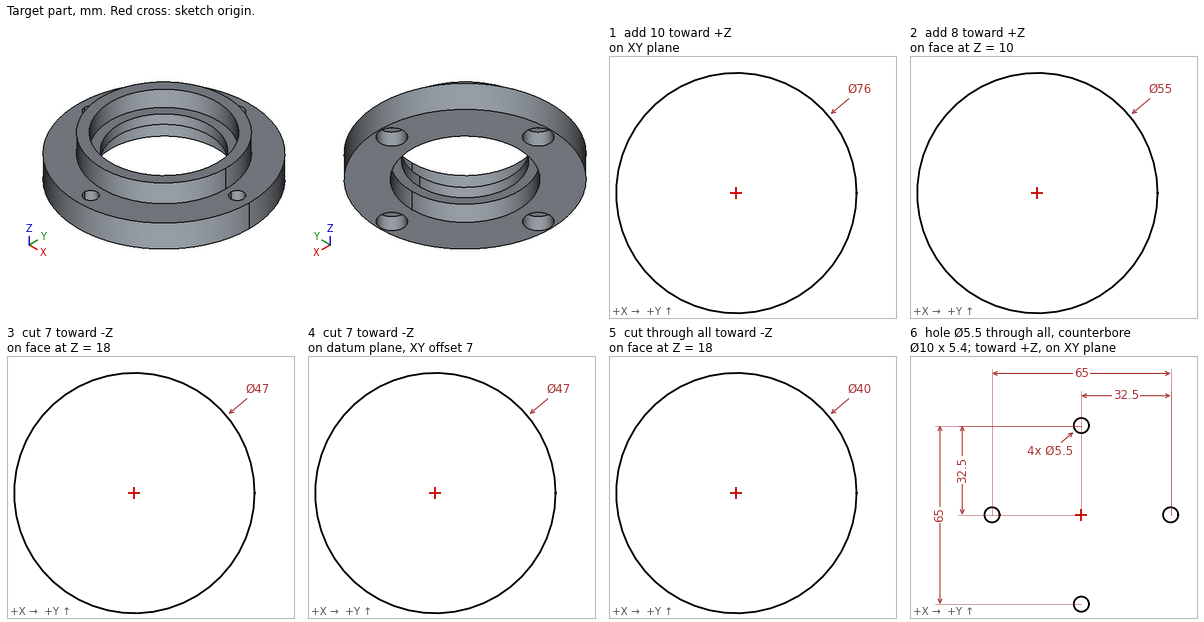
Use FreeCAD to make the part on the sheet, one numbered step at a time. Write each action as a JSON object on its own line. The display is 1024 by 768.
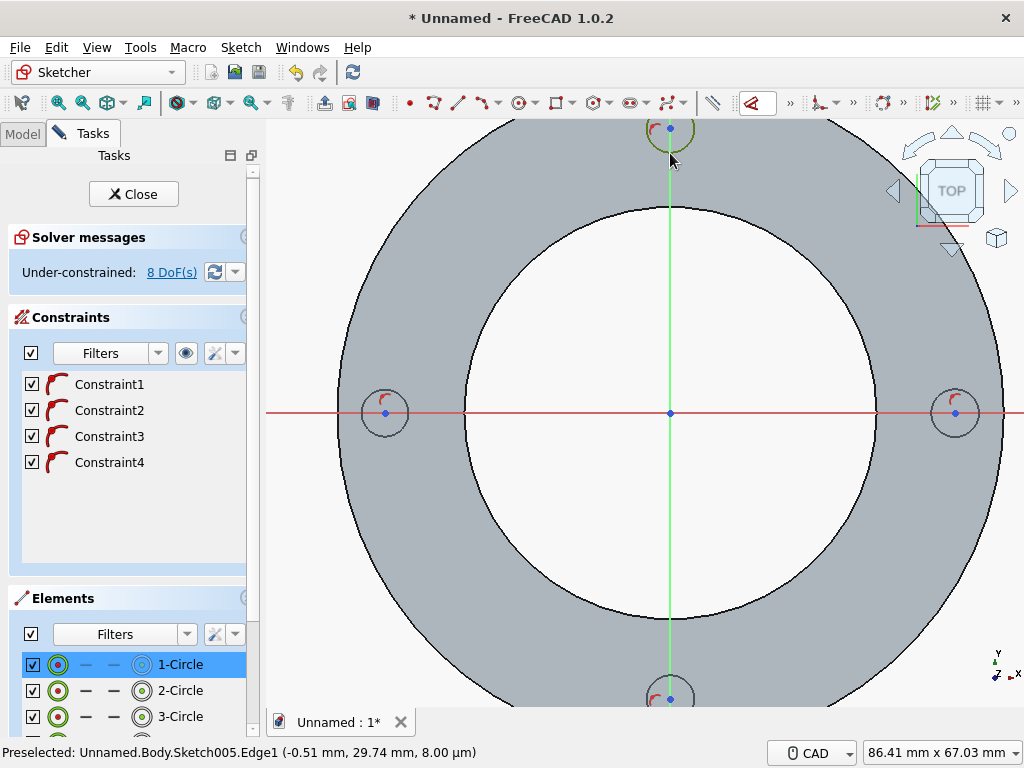
{"action": "scroll", "coordinate": [385, 413], "scroll_direction": "down", "scroll_amount": 2}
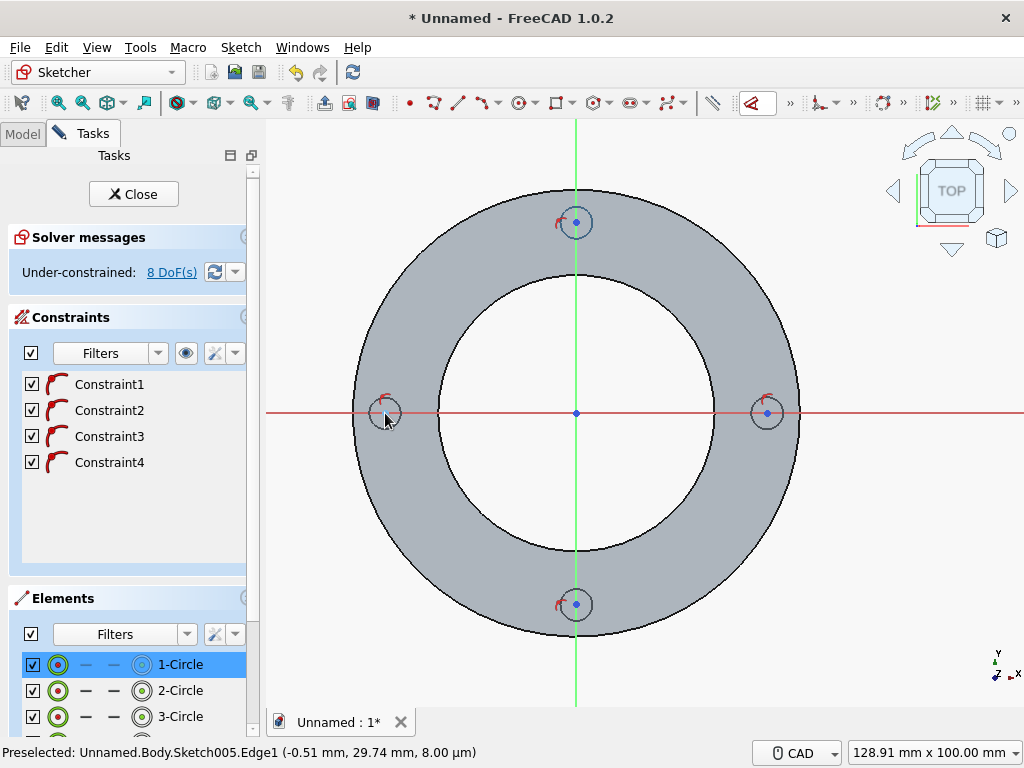
{"action": "left_click", "coordinate": [778, 402]}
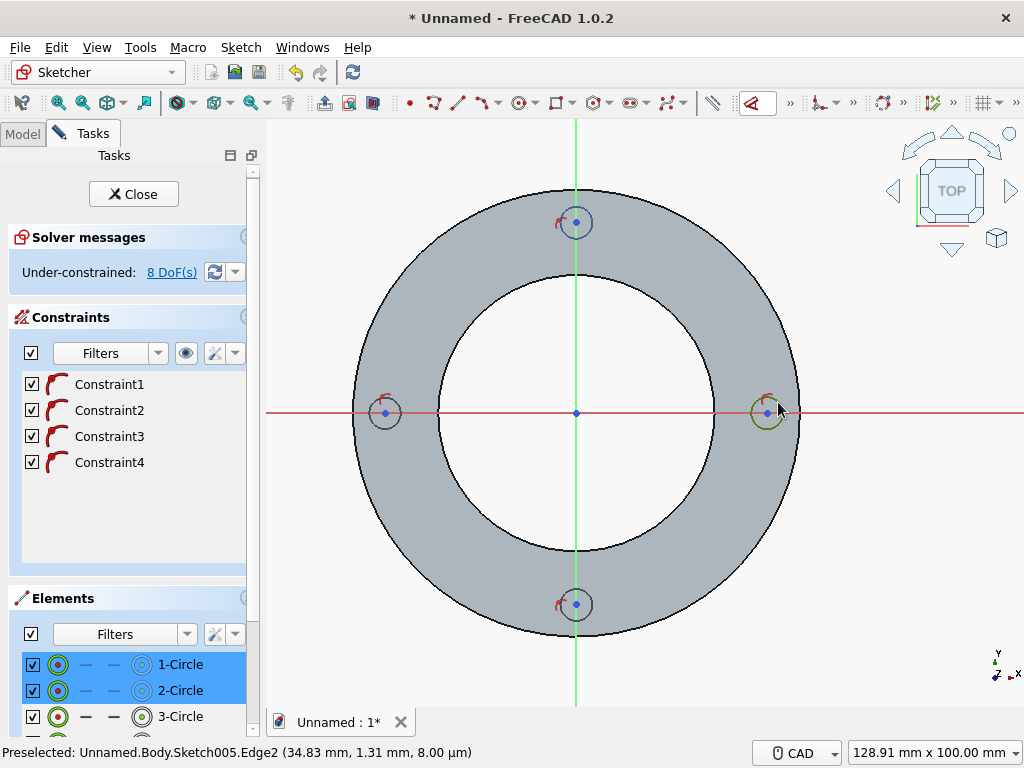
{"action": "scroll", "coordinate": [588, 594], "scroll_direction": "up", "scroll_amount": 2}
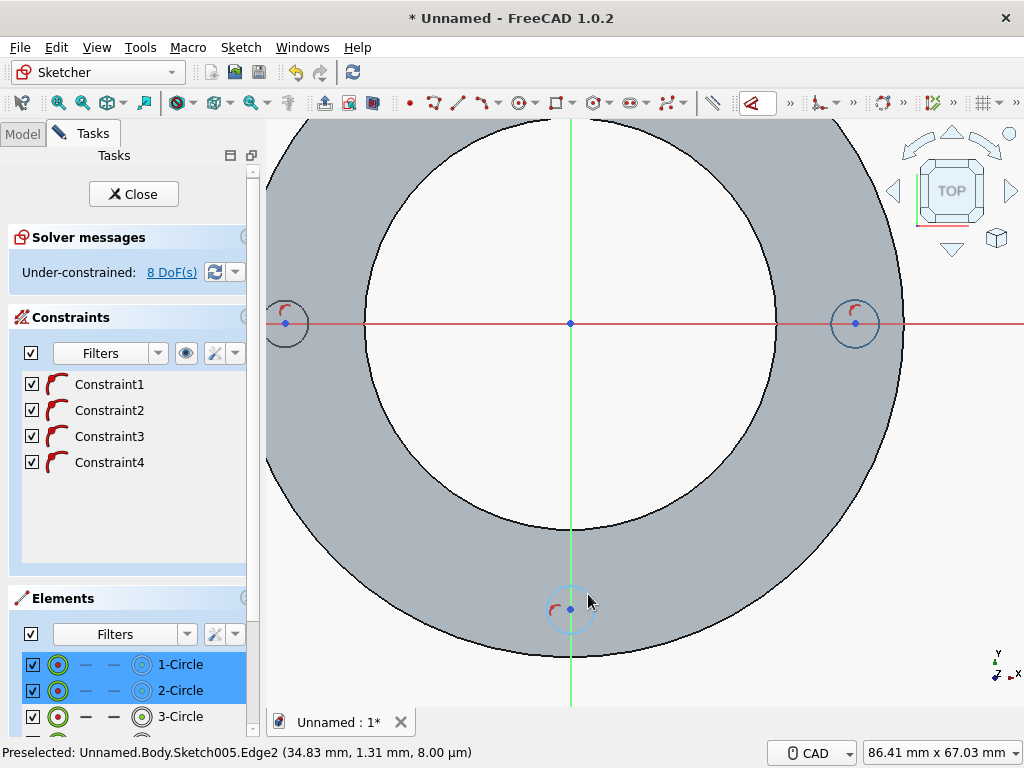
{"action": "left_click", "coordinate": [587, 593]}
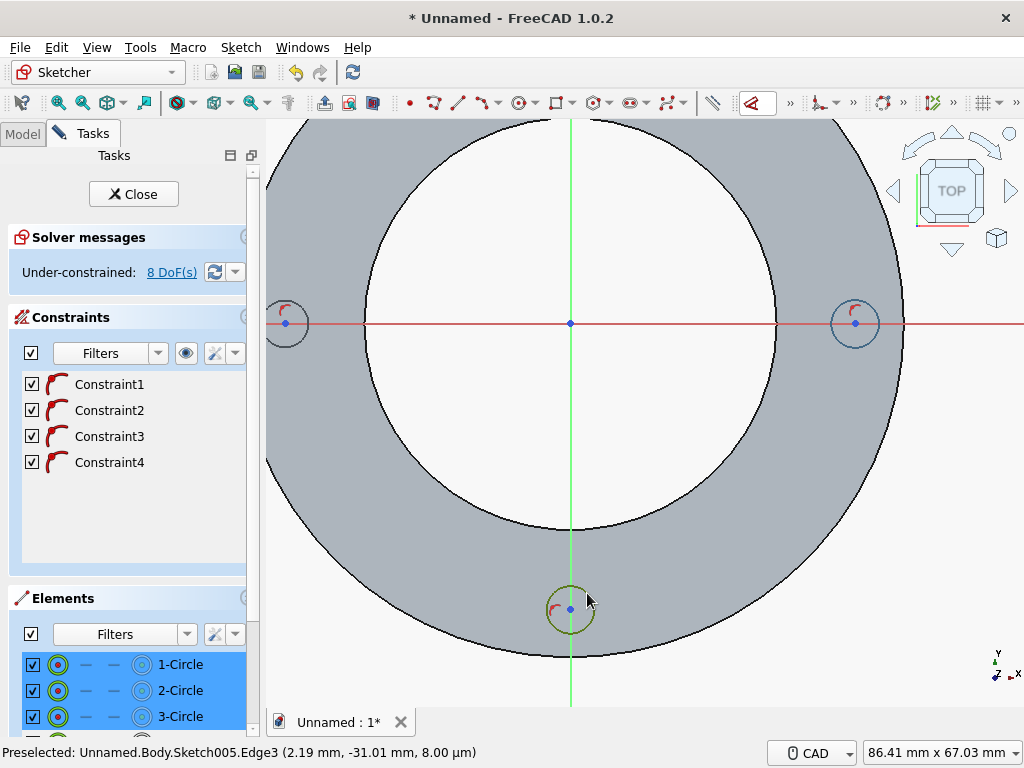
{"action": "left_click", "coordinate": [302, 307]}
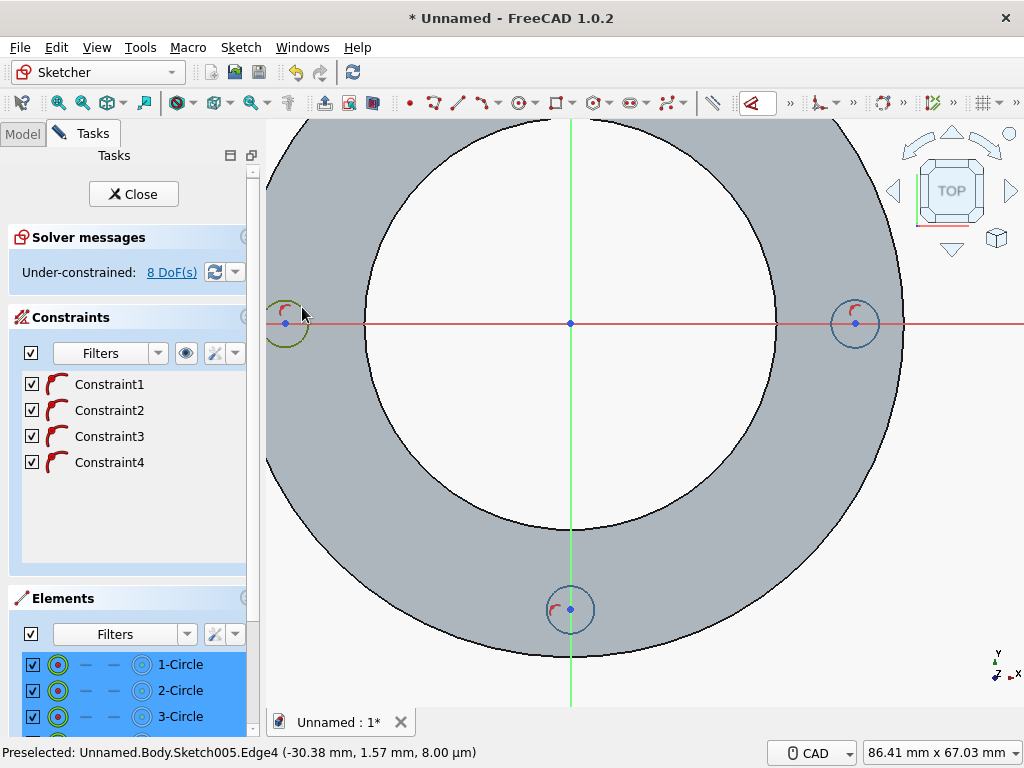
{"action": "key", "text": "e"}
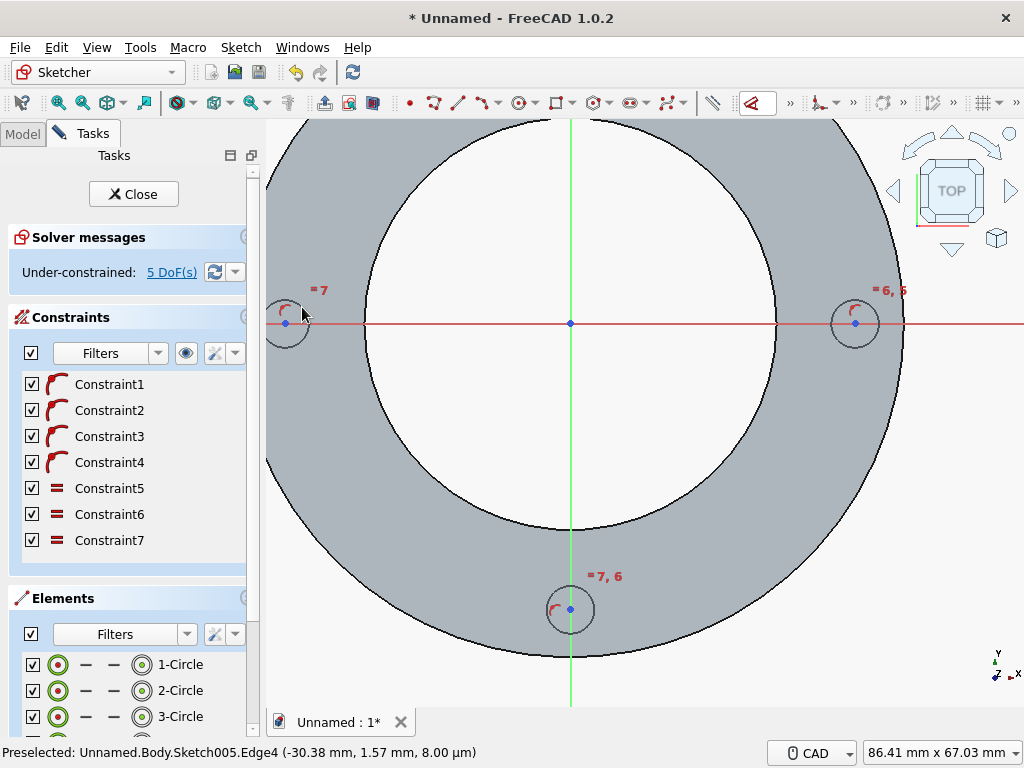
{"action": "scroll", "coordinate": [589, 594], "scroll_direction": "down", "scroll_amount": 2}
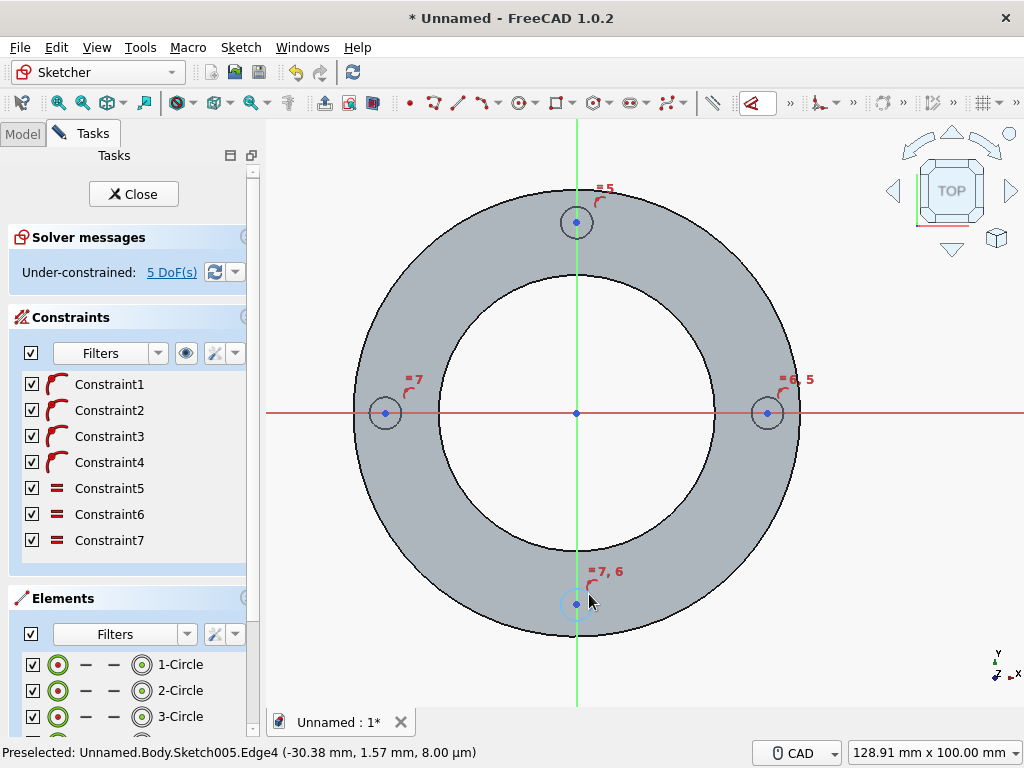
{"action": "scroll", "coordinate": [588, 211], "scroll_direction": "up", "scroll_amount": 2}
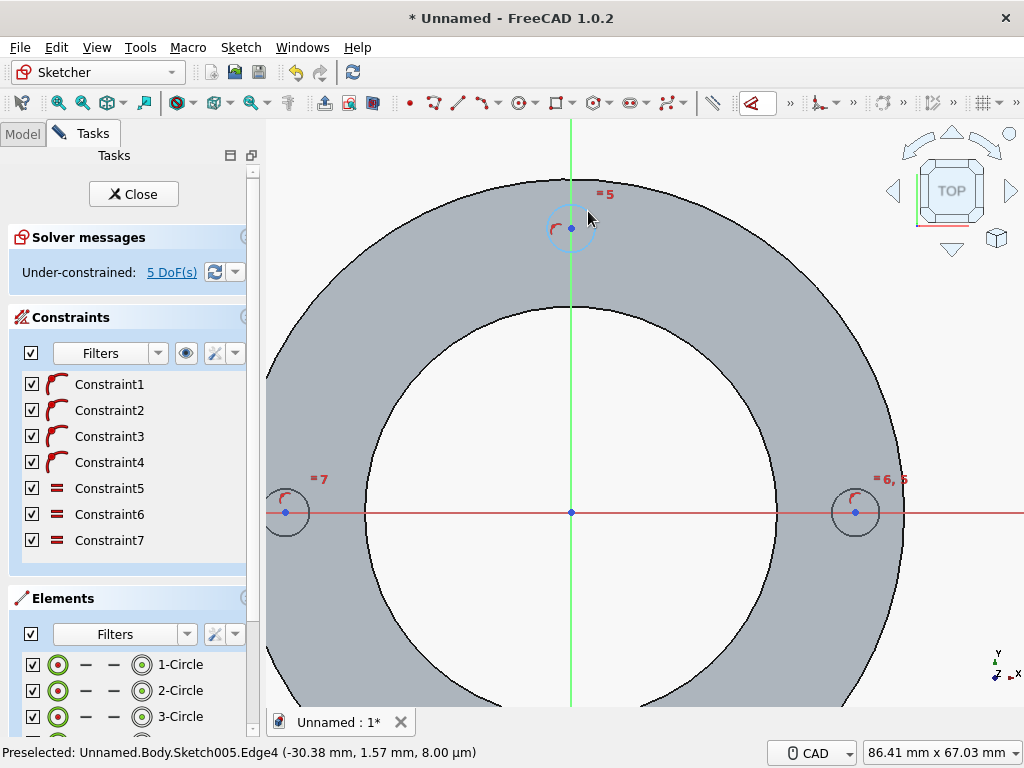
{"action": "left_click", "coordinate": [588, 212]}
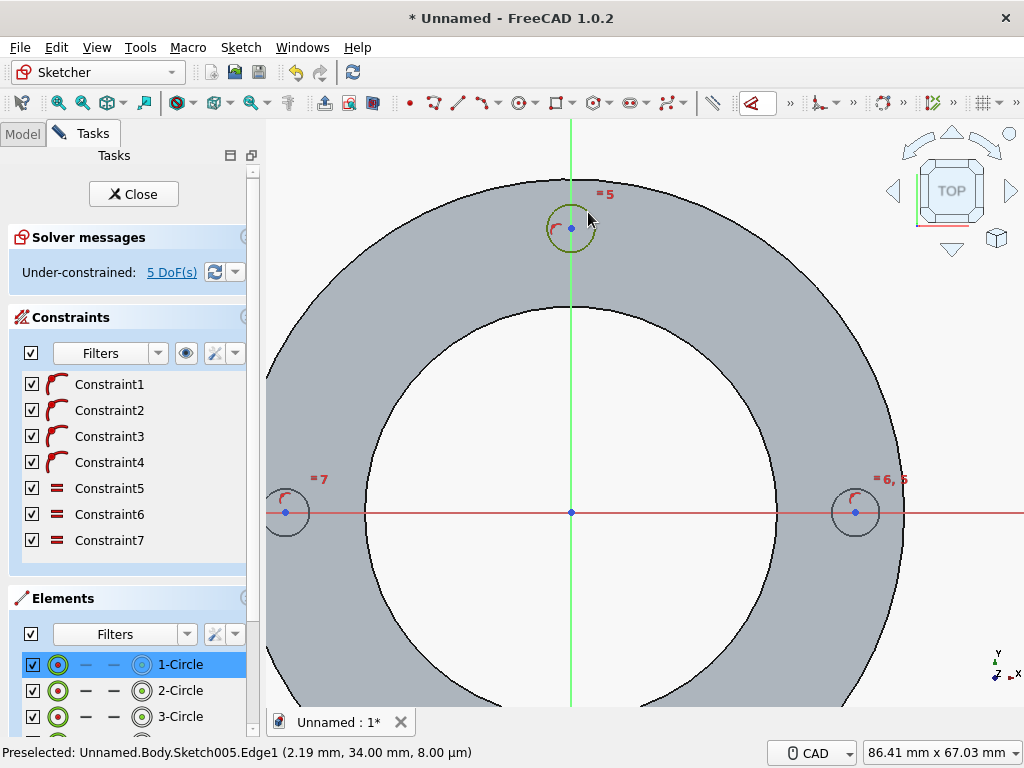
{"action": "left_click", "coordinate": [770, 104]}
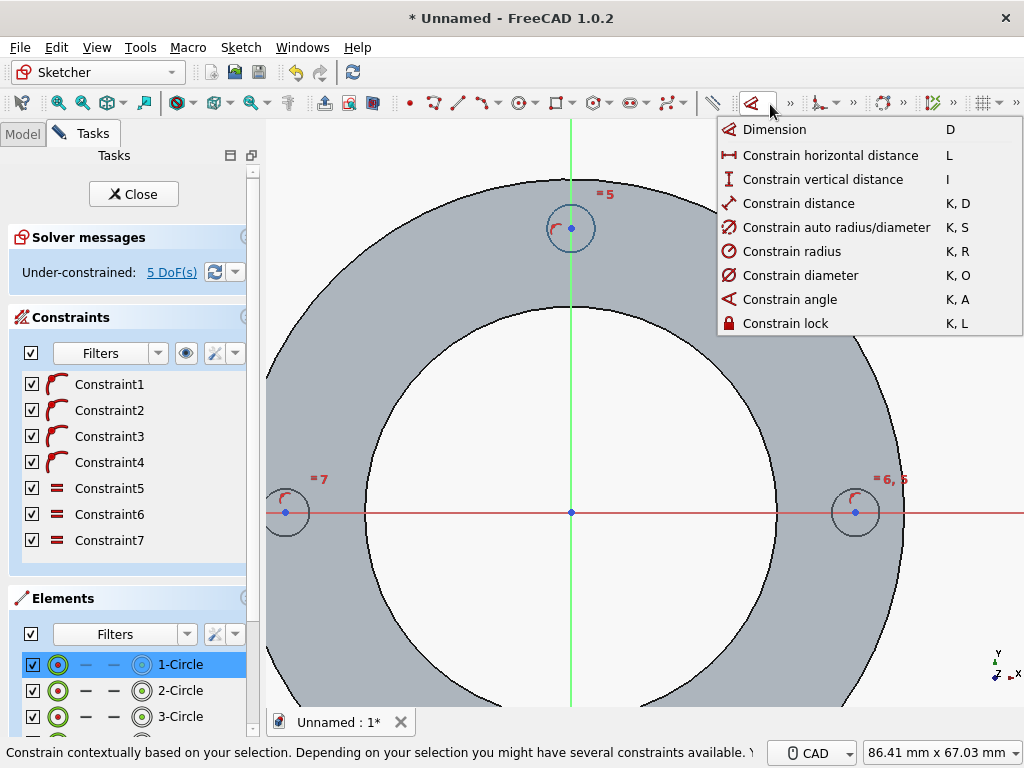
{"action": "left_click", "coordinate": [870, 275]}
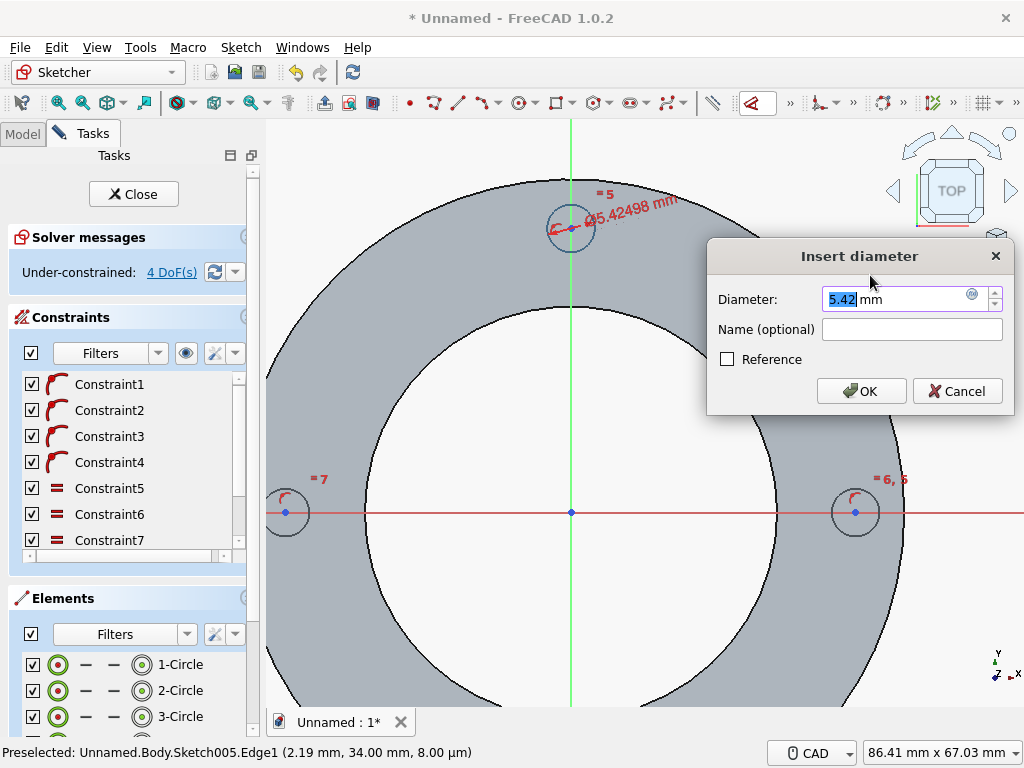
{"action": "type", "text": "5.5"}
{"action": "key", "text": "Return"}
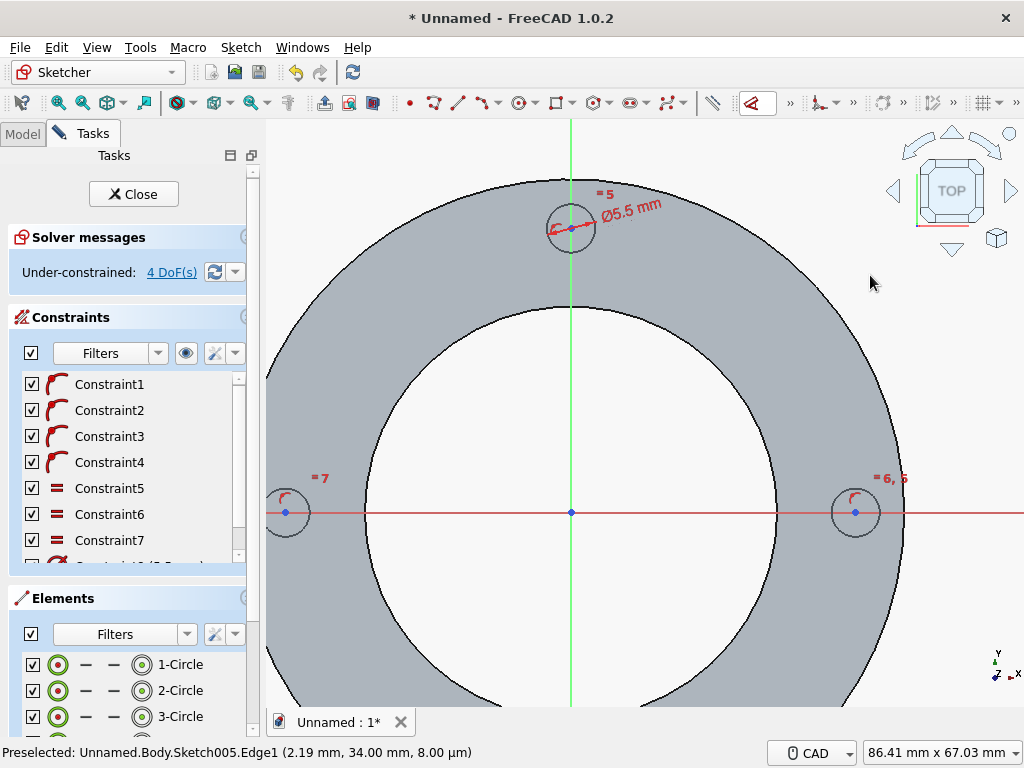
{"action": "left_click", "coordinate": [571, 228]}